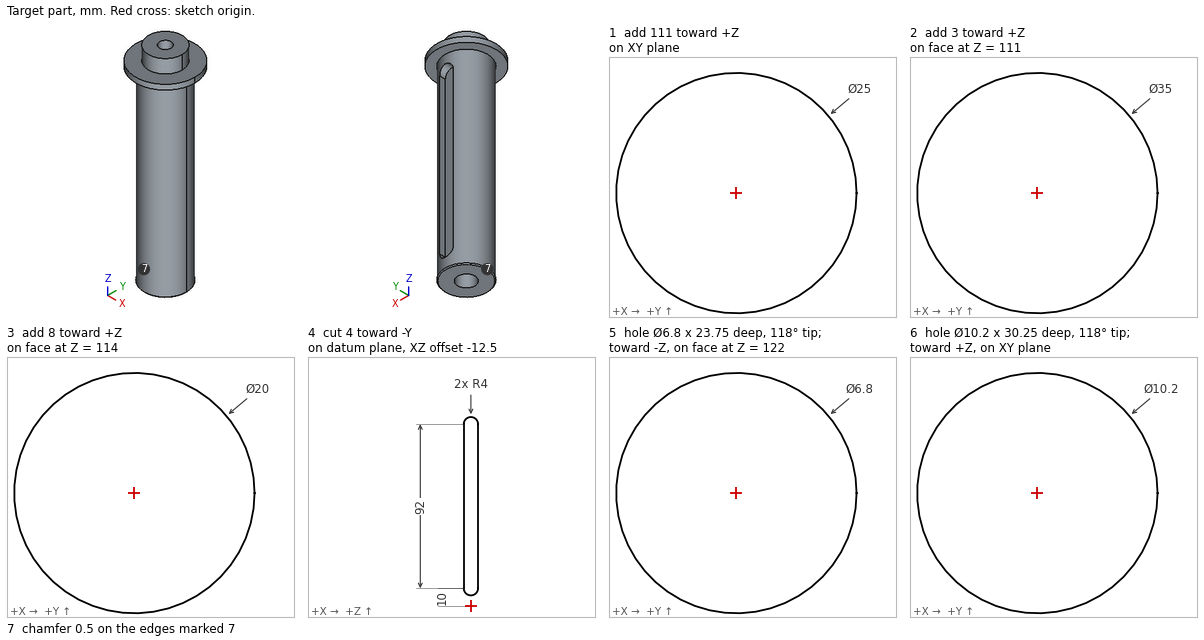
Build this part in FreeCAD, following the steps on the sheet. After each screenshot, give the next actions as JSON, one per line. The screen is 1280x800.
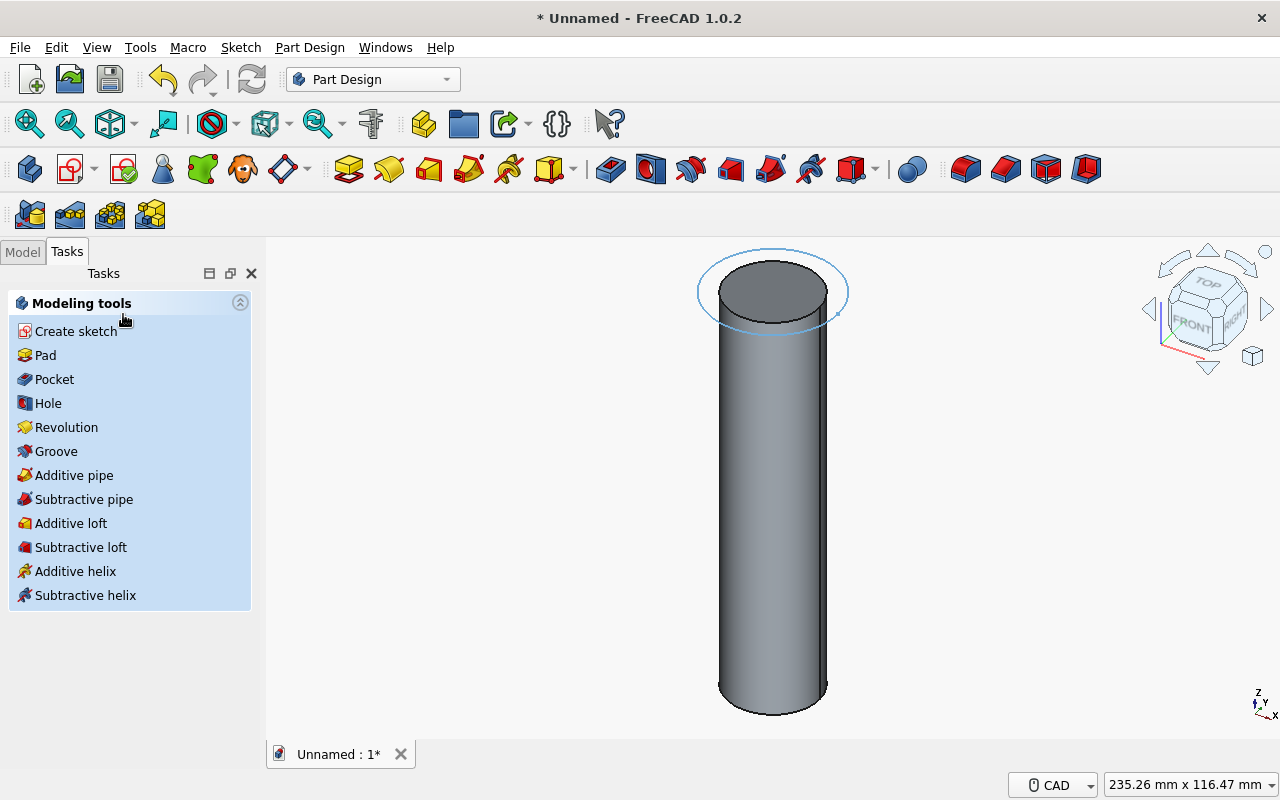
{"action": "left_click", "coordinate": [350, 170]}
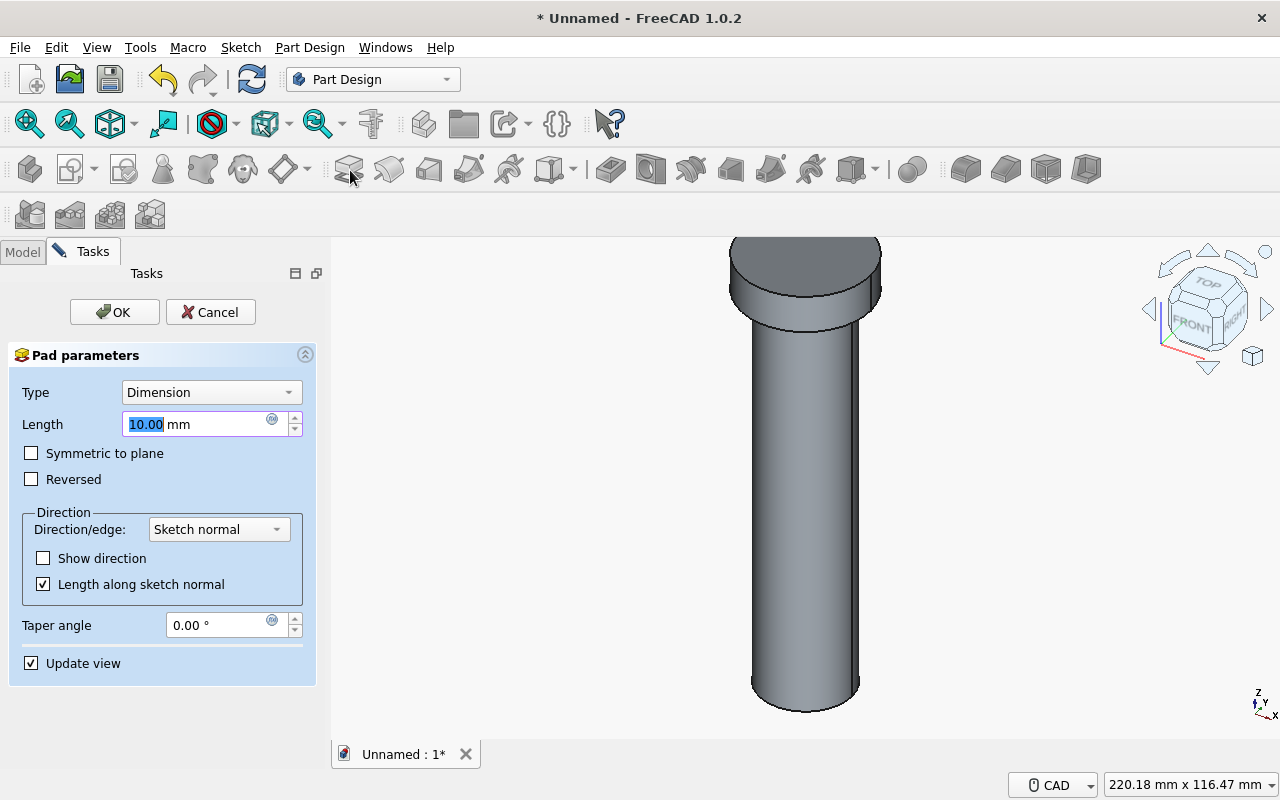
{"action": "type", "text": "3"}
{"action": "key", "text": "Tab"}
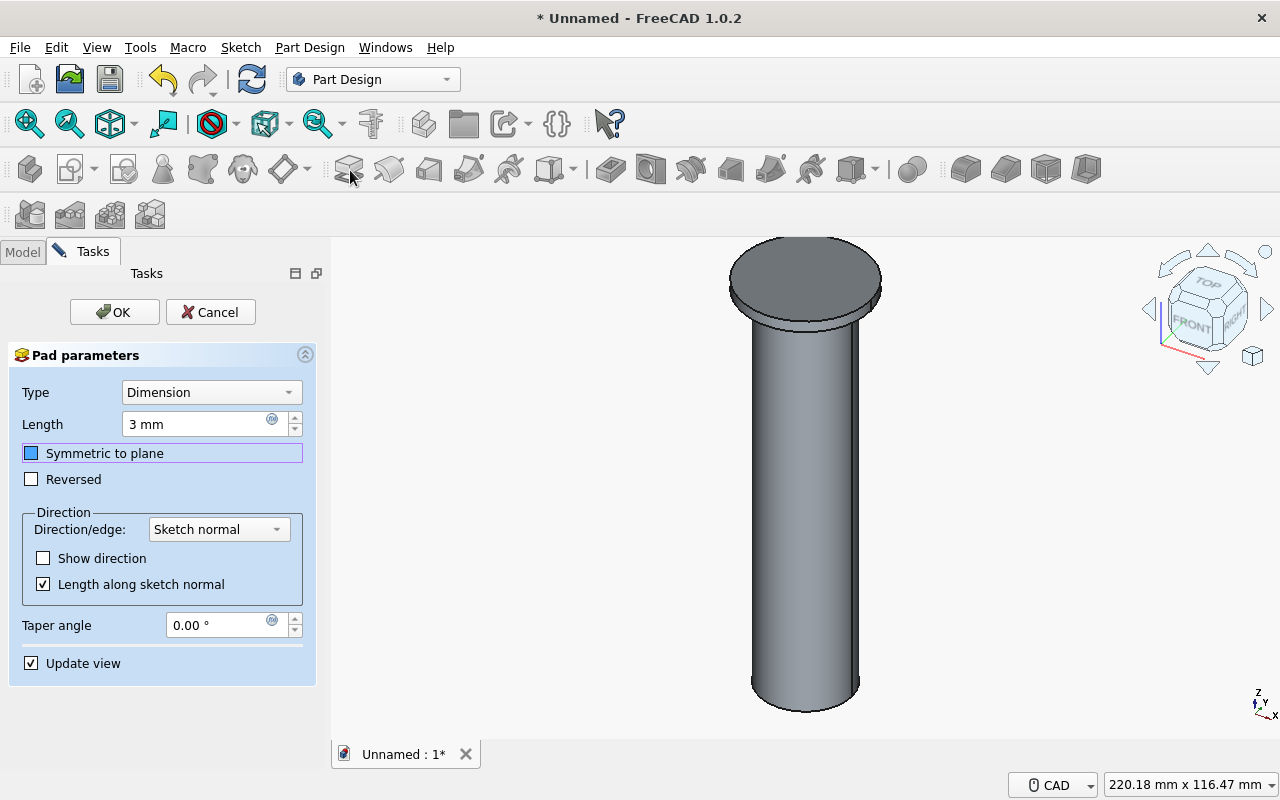
{"action": "left_click", "coordinate": [115, 312]}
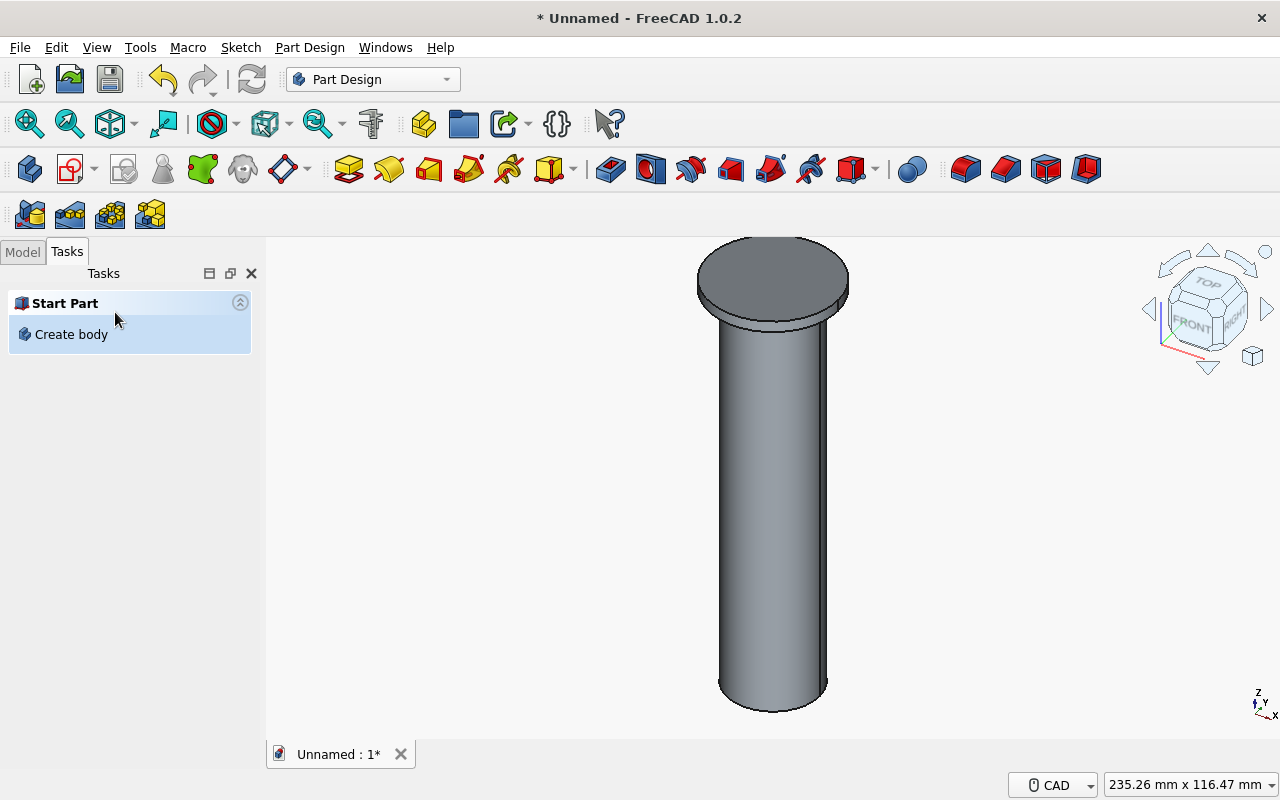
{"action": "left_click", "coordinate": [30, 124]}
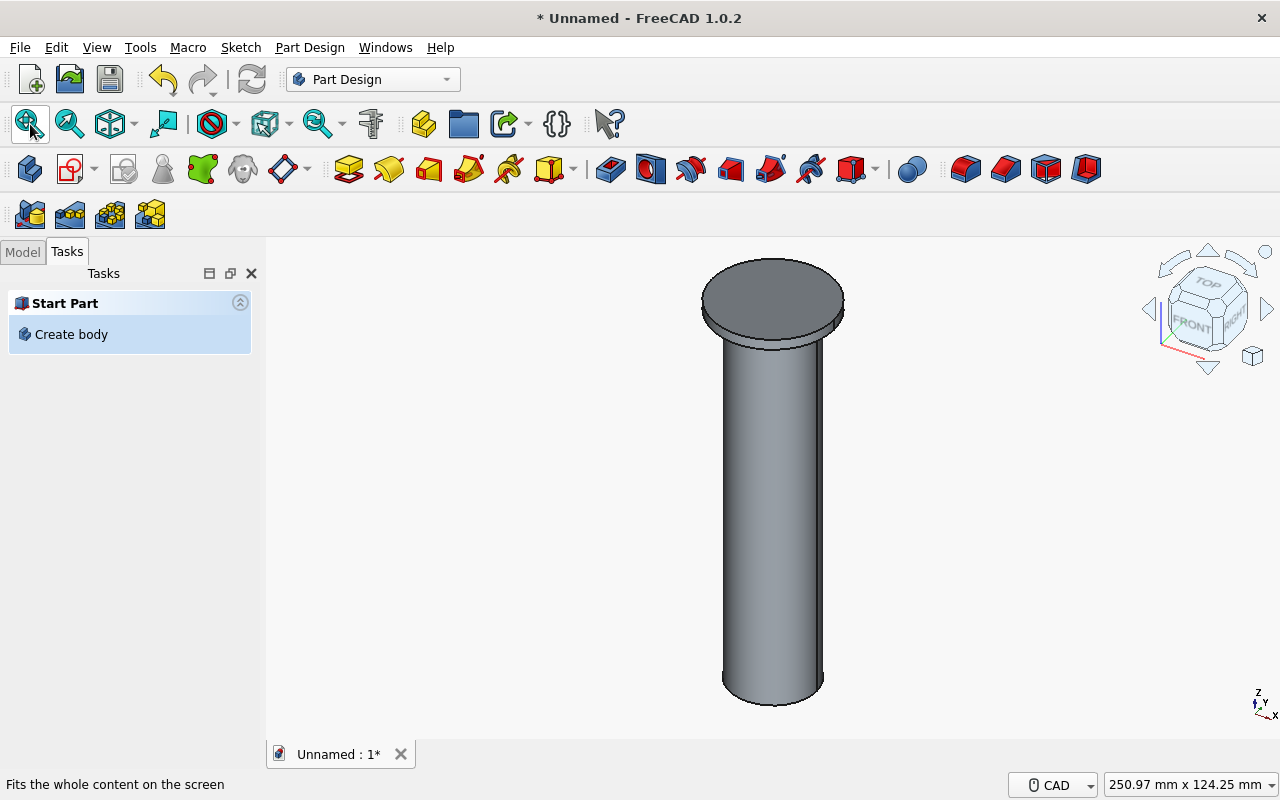
{"action": "left_click", "coordinate": [773, 298]}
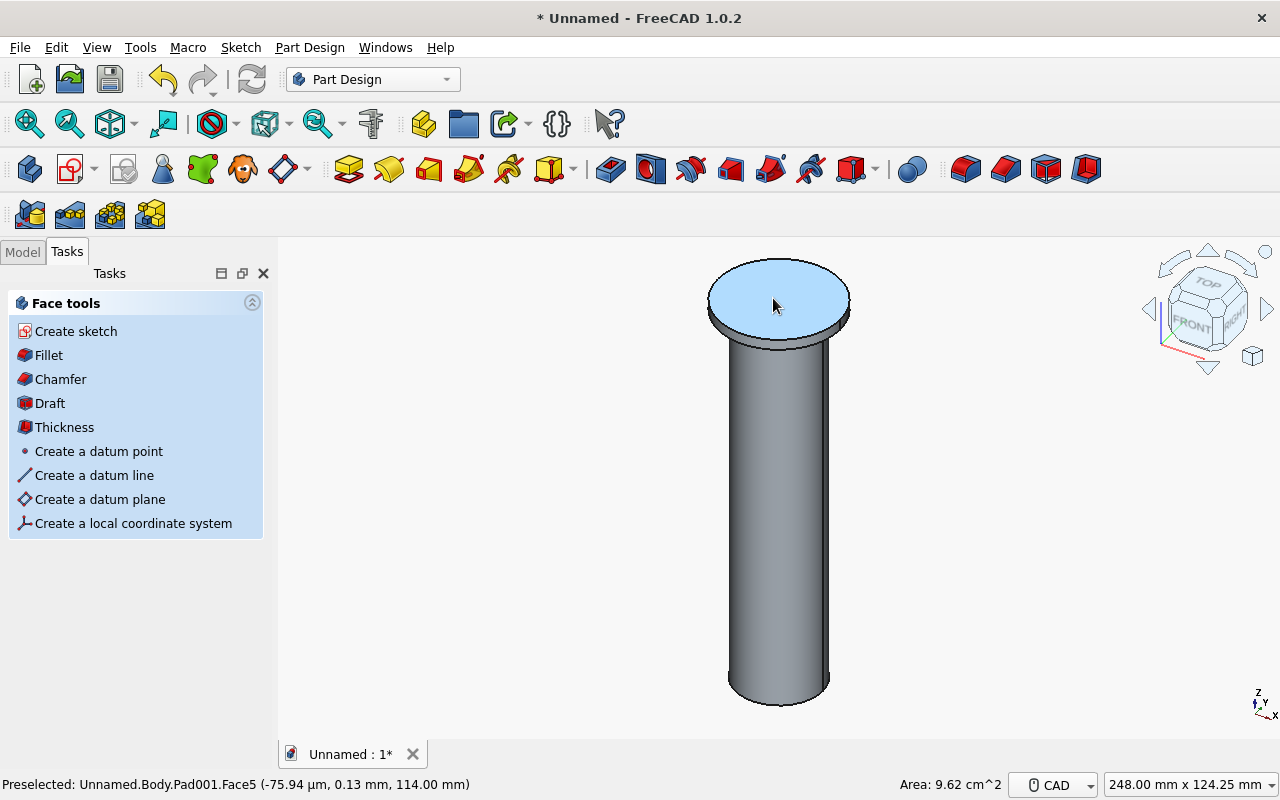
{"action": "left_click", "coordinate": [70, 170]}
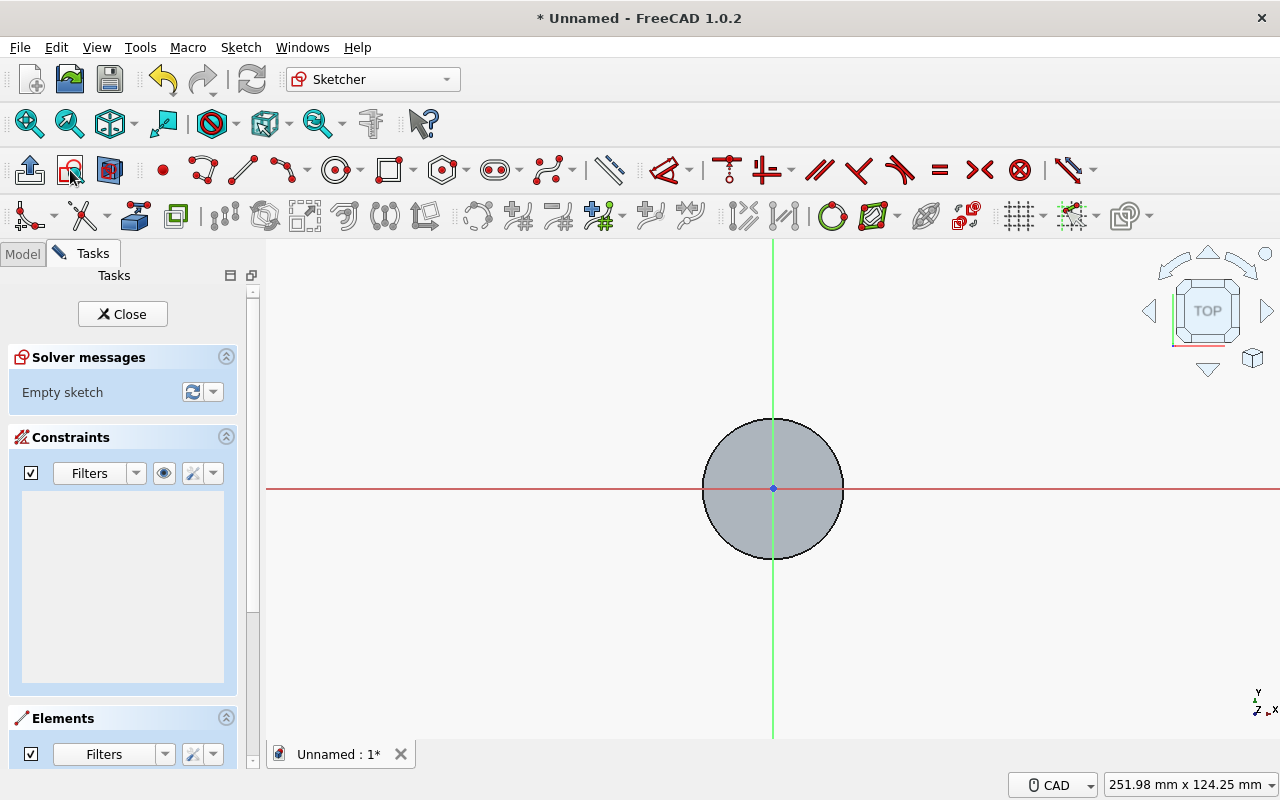
{"action": "scroll", "coordinate": [795, 489], "scroll_direction": "up", "scroll_amount": 7}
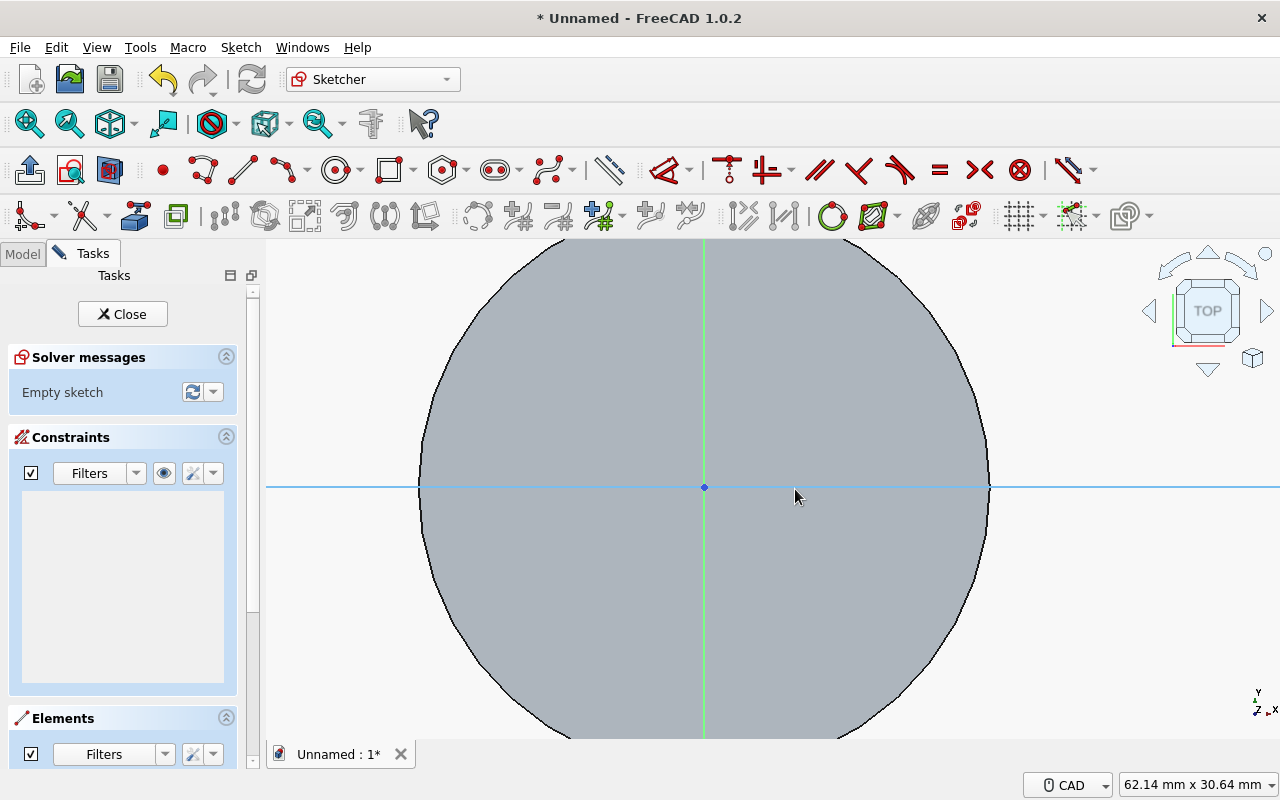
{"action": "left_click", "coordinate": [336, 170]}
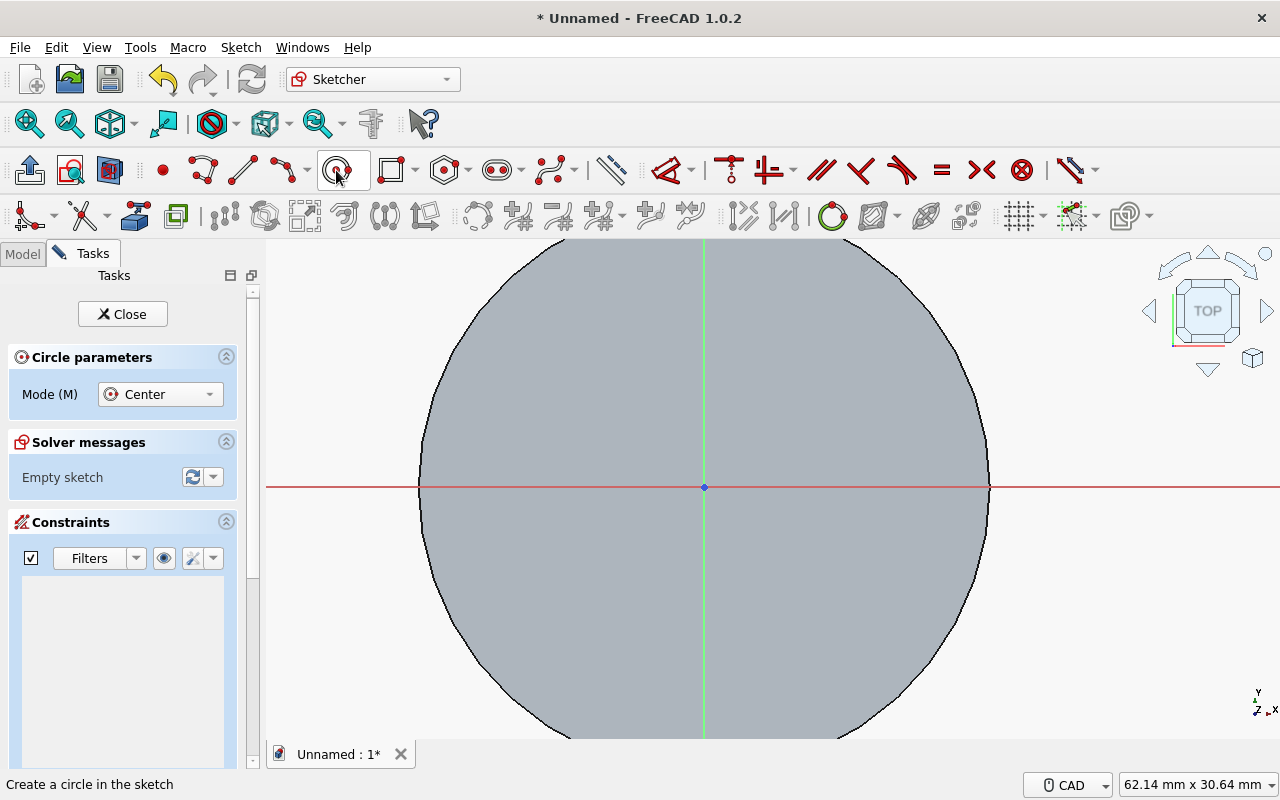
{"action": "left_click", "coordinate": [704, 487]}
{"action": "mouse_move", "coordinate": [820, 372]}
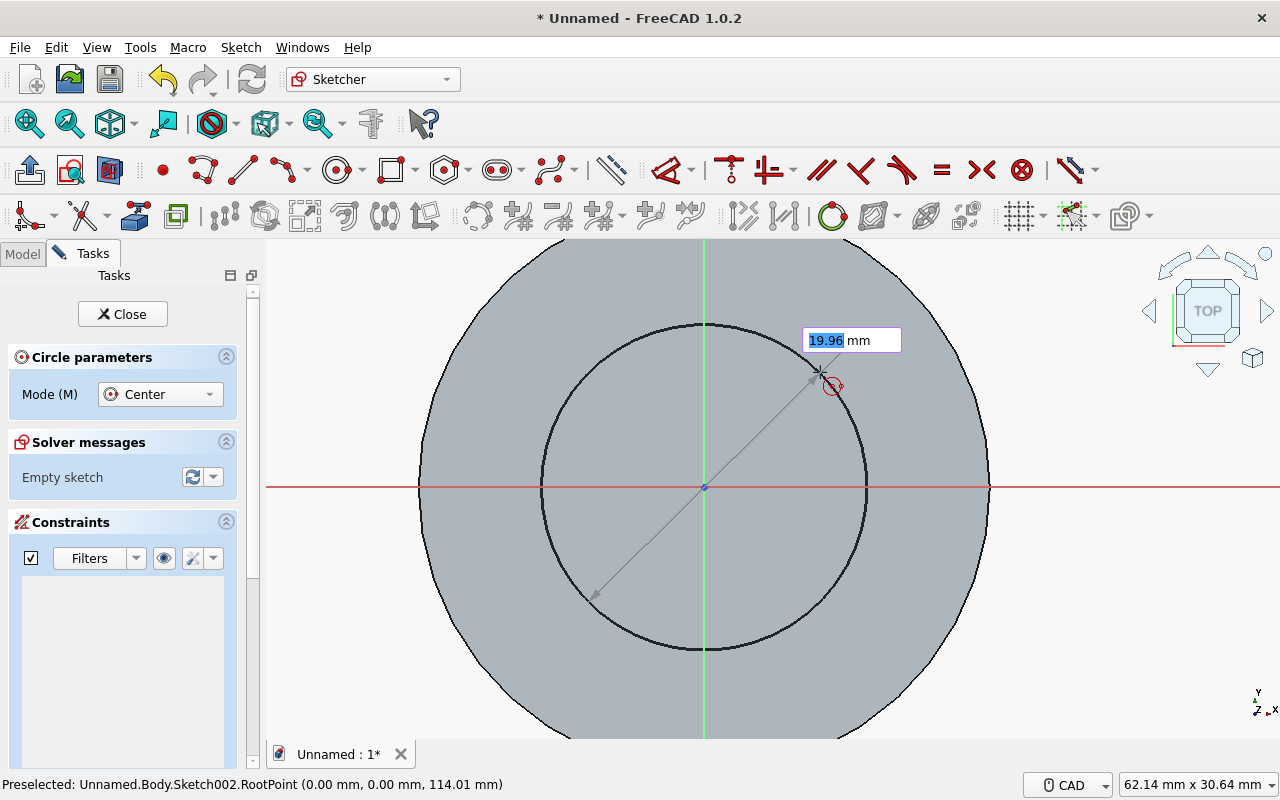
{"action": "type", "text": "20"}
{"action": "key", "text": "Return"}
{"action": "key", "text": "Escape"}